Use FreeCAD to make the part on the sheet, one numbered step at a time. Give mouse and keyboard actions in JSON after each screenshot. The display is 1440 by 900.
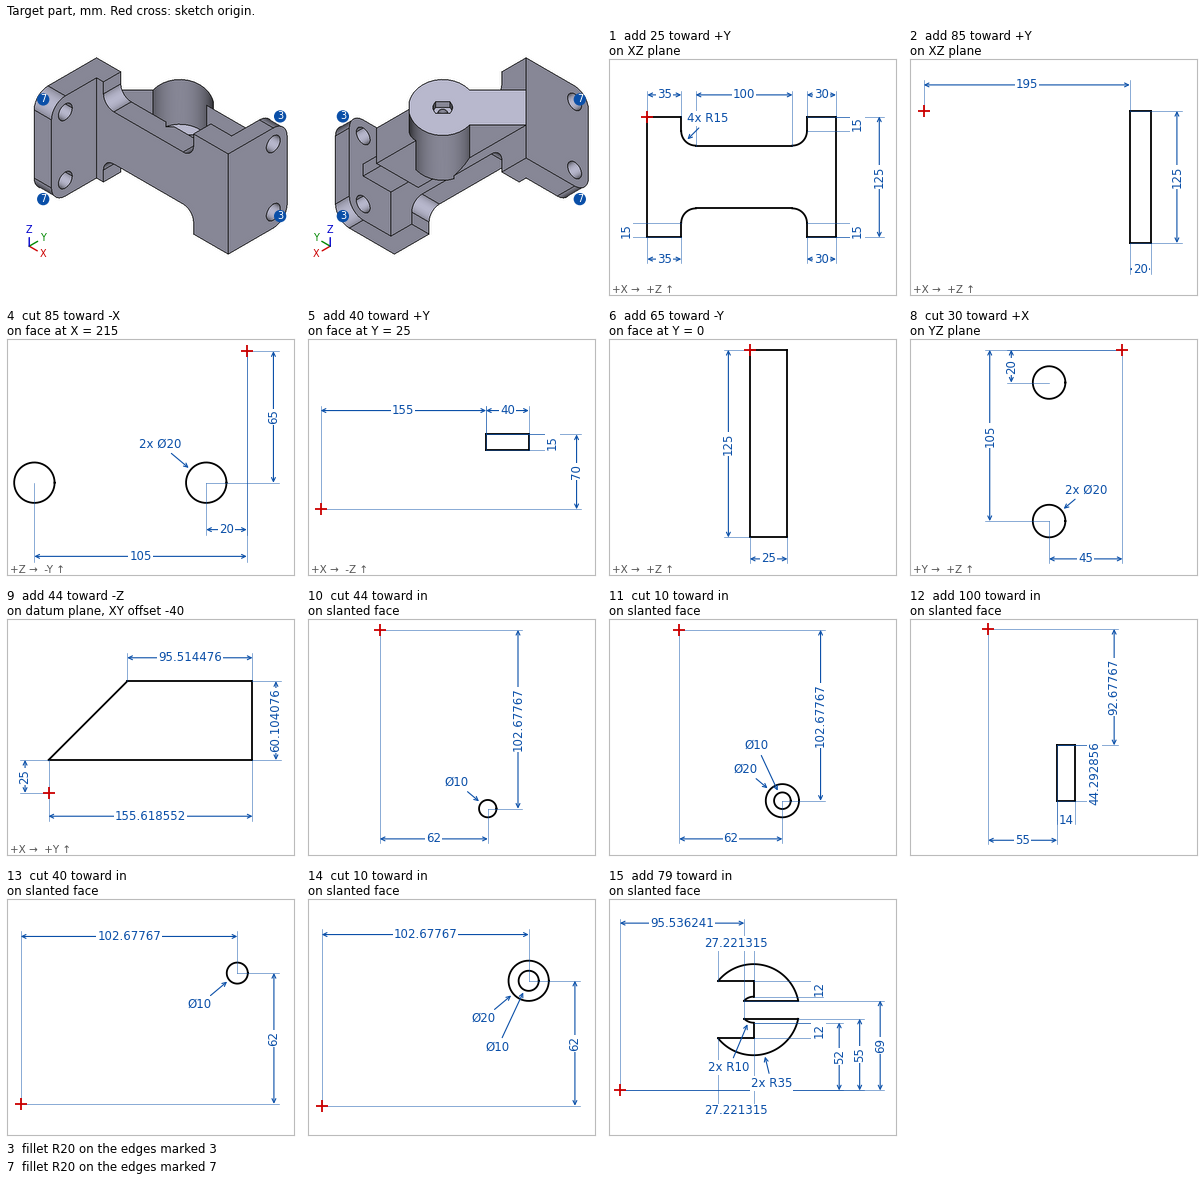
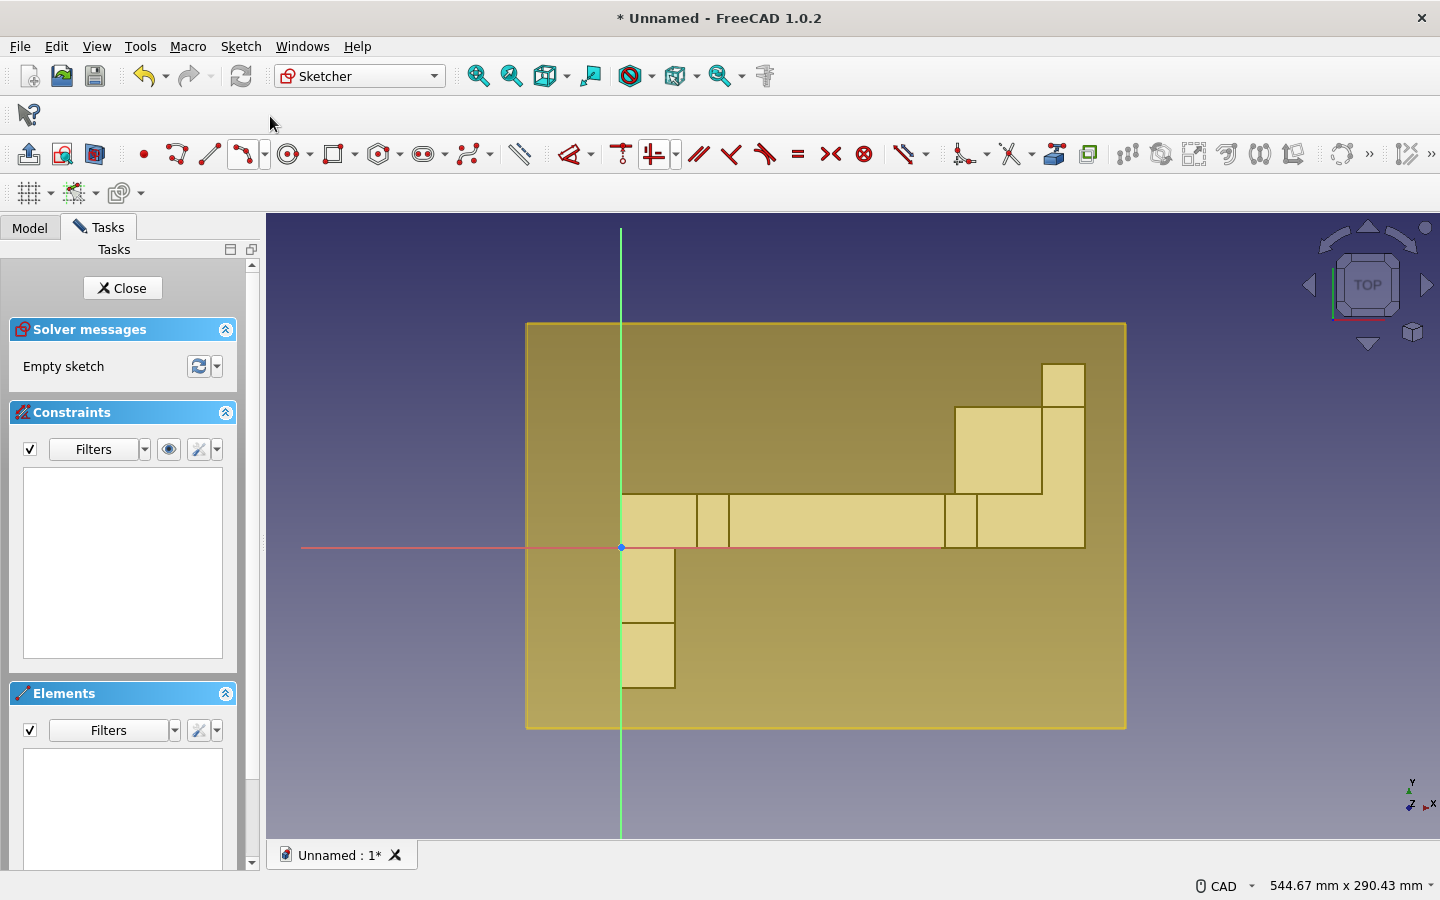
{"action": "scroll", "coordinate": [793, 399], "scroll_direction": "up", "scroll_amount": 4}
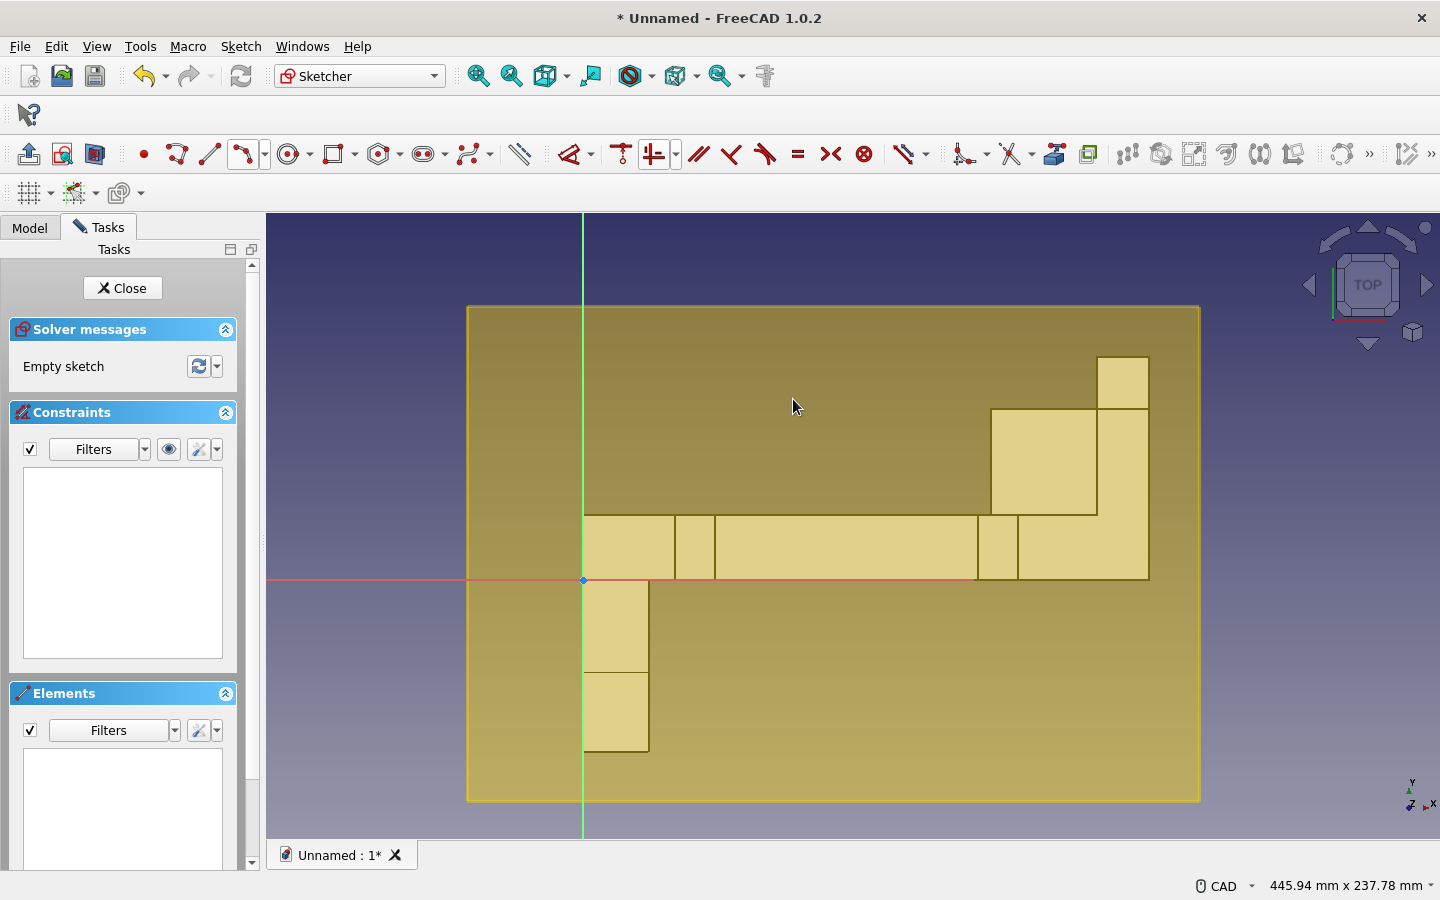
{"action": "left_click", "coordinate": [177, 154]}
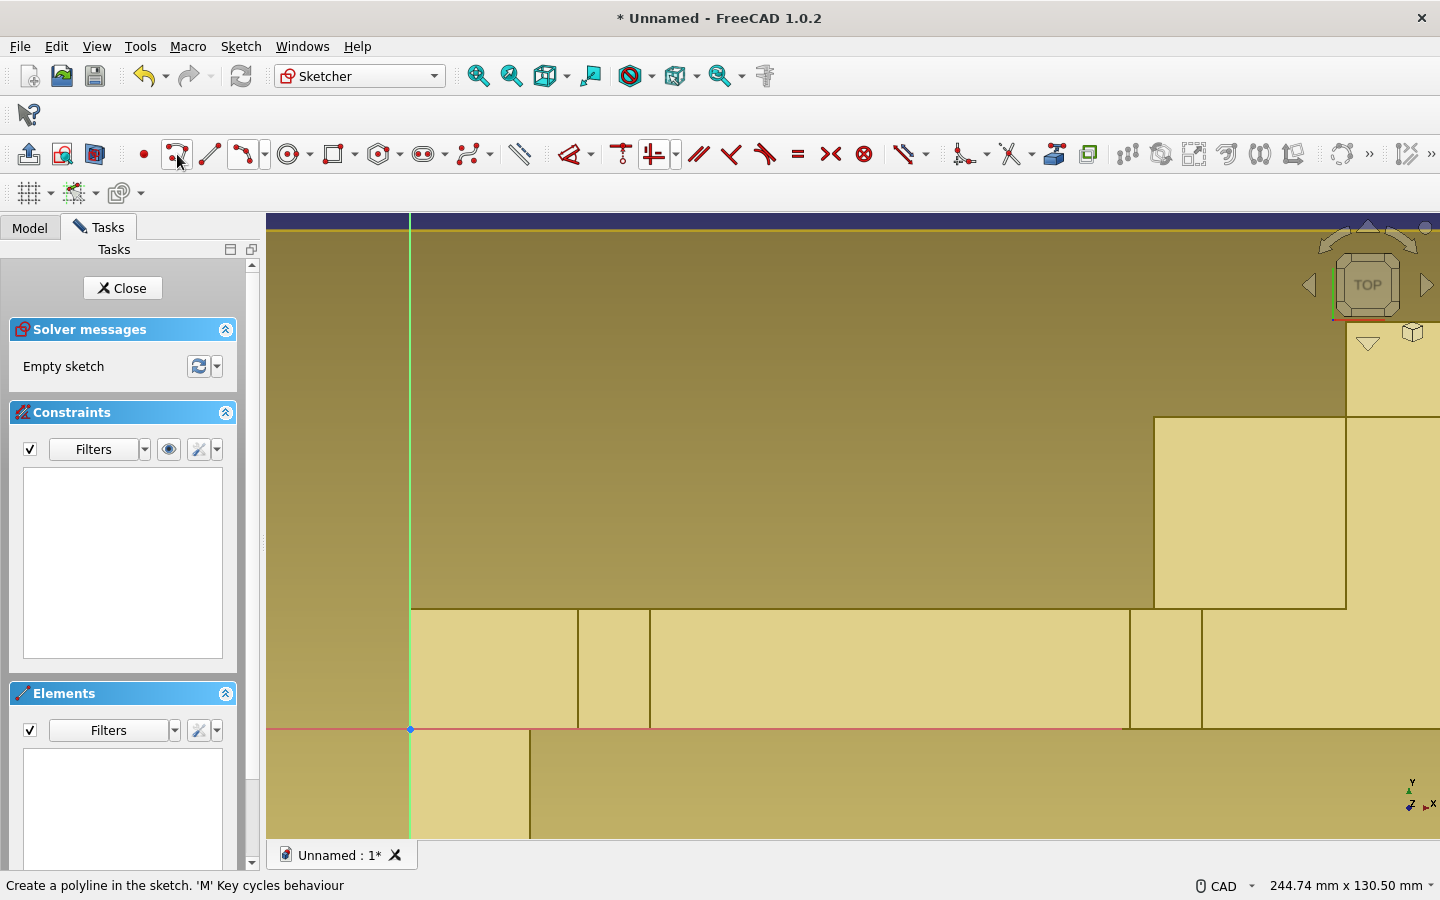
{"action": "left_click", "coordinate": [410, 609]}
{"action": "left_click", "coordinate": [1157, 609]}
{"action": "left_click", "coordinate": [1157, 321]}
{"action": "left_click", "coordinate": [699, 321]}
{"action": "left_click", "coordinate": [410, 610]}
{"action": "key", "text": "Escape"}
{"action": "key", "text": "Escape"}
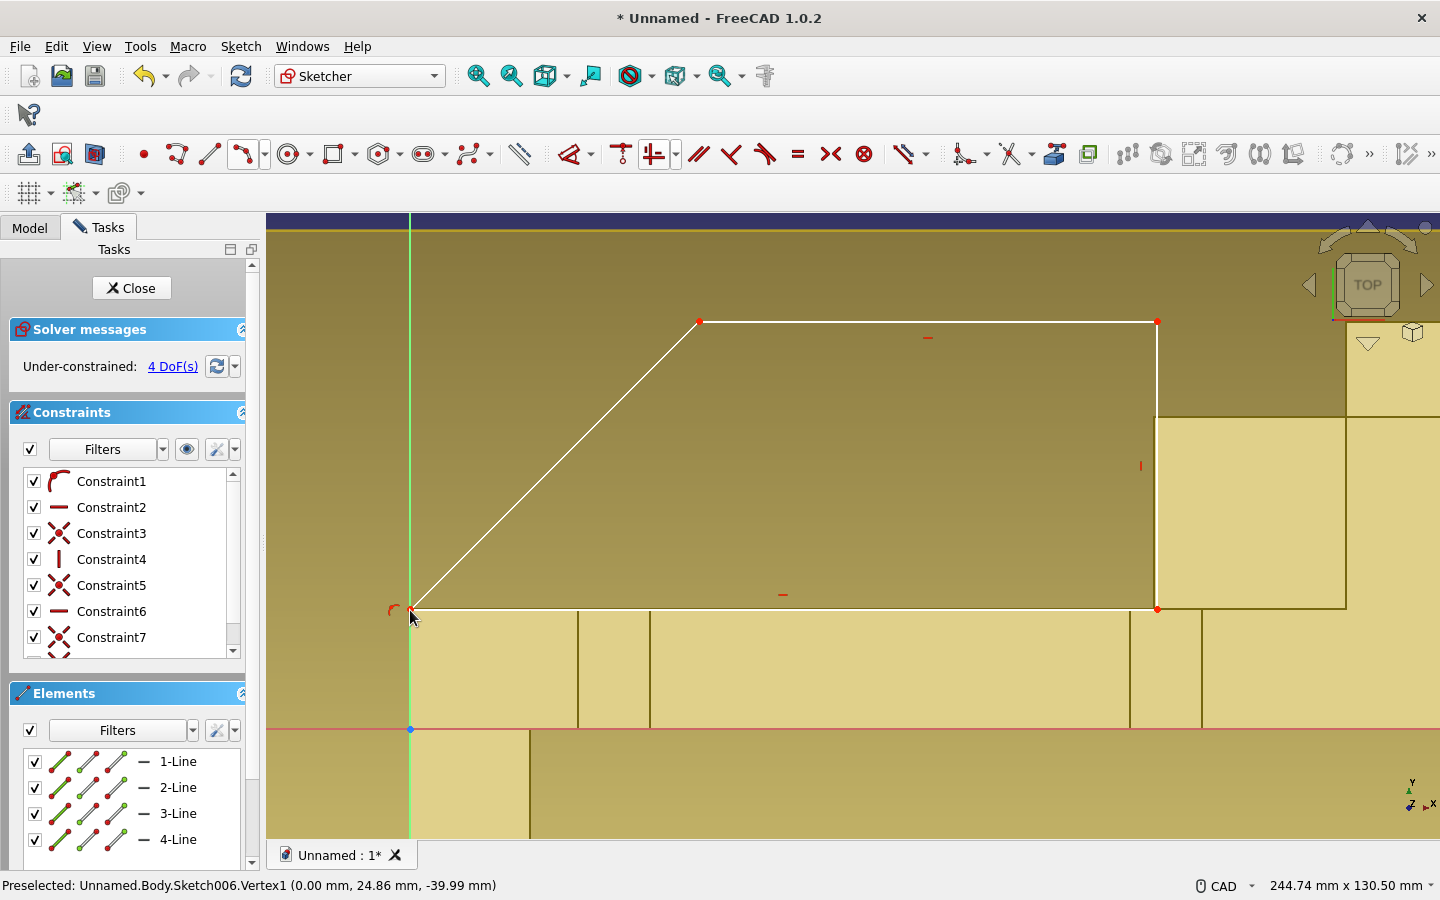
{"action": "left_click", "coordinate": [568, 154]}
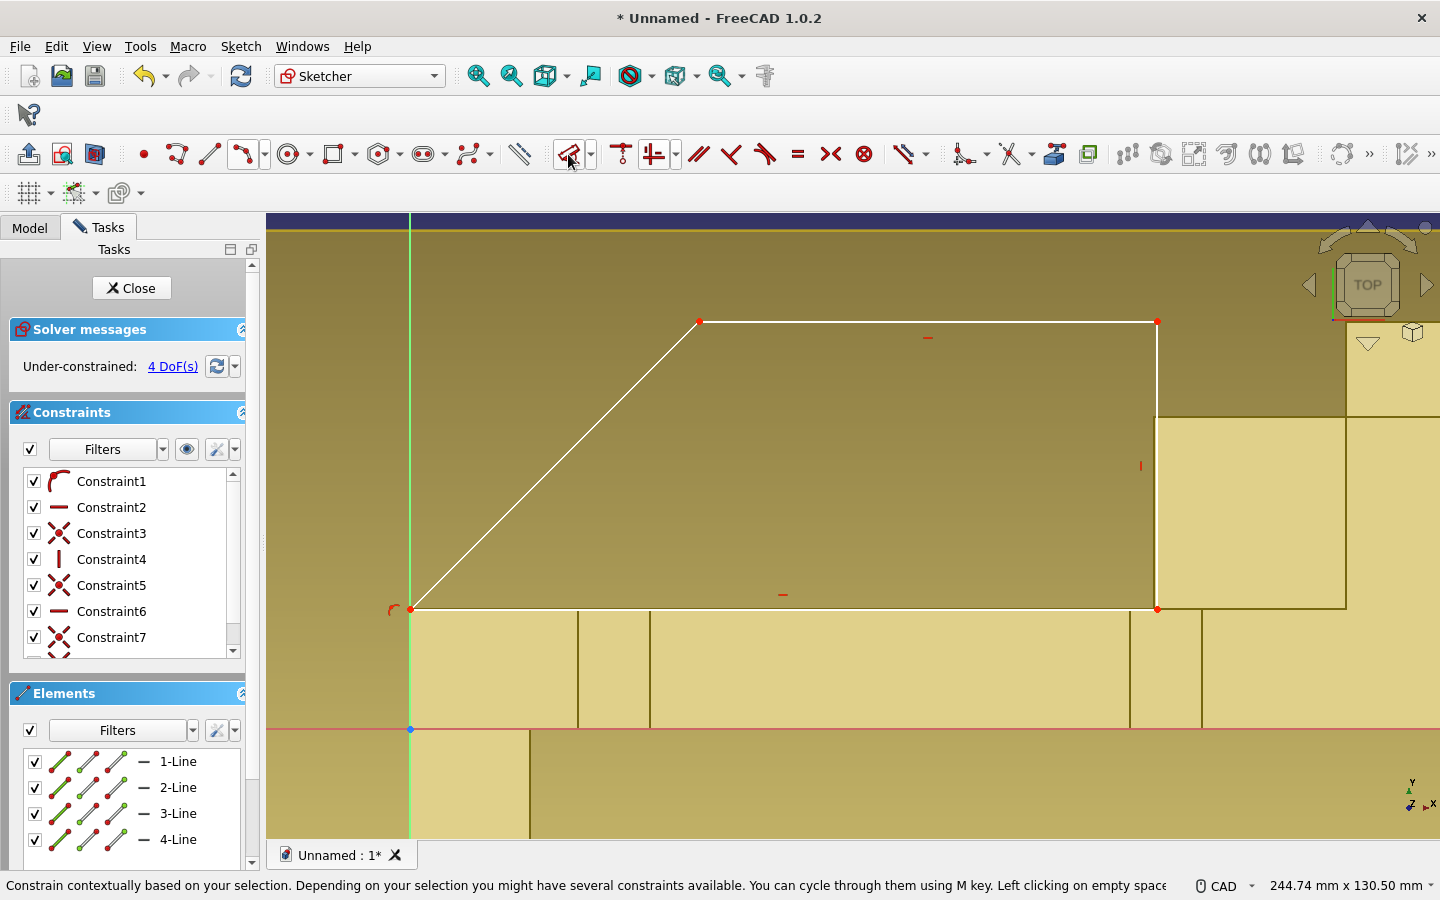
{"action": "left_click", "coordinate": [410, 610]}
{"action": "left_click", "coordinate": [376, 670]}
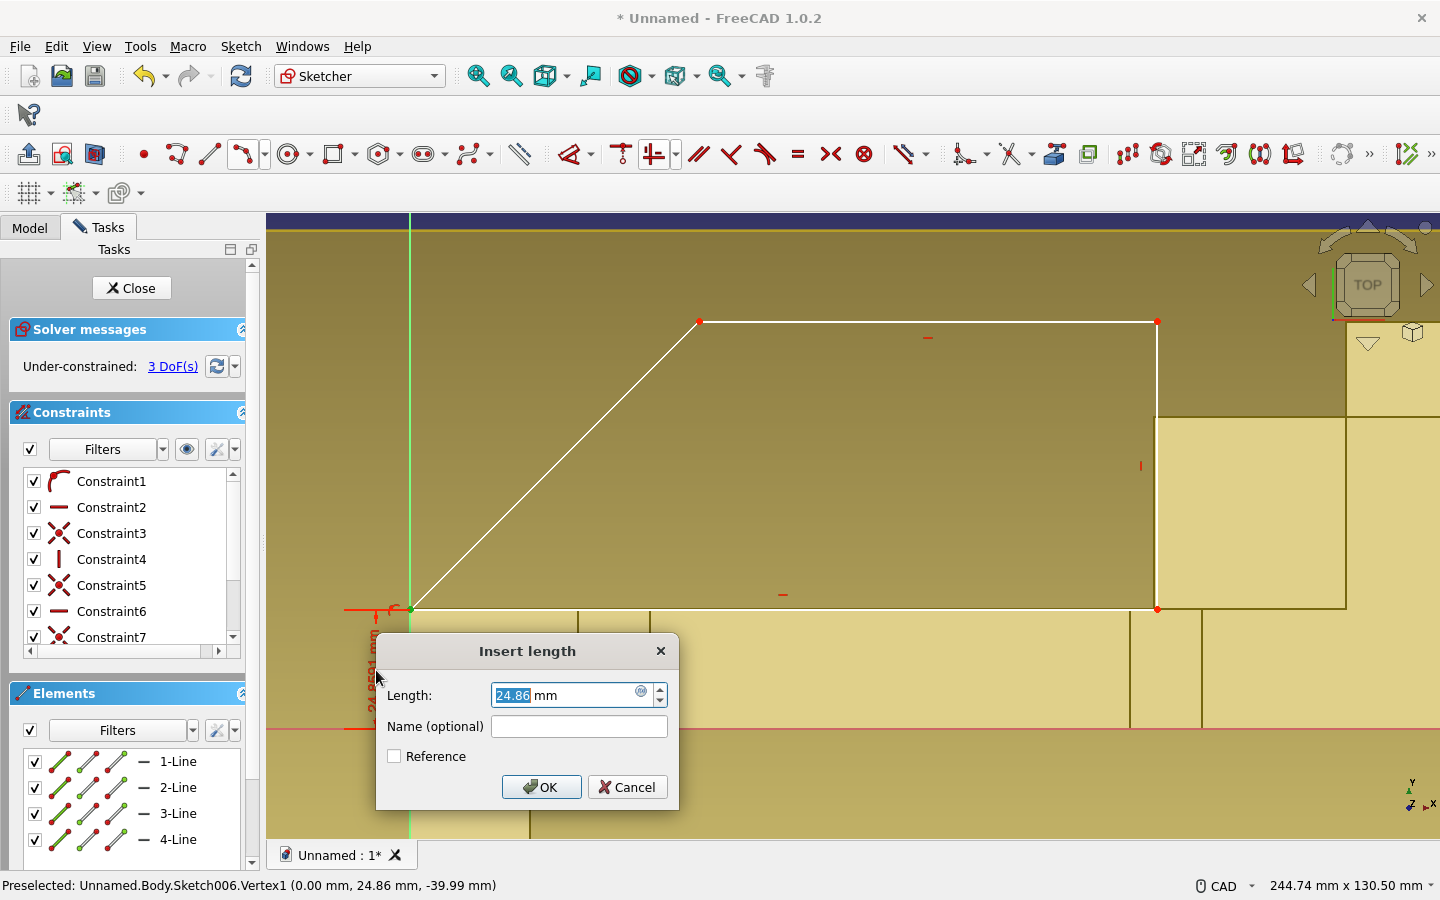
{"action": "type", "text": "25"}
{"action": "key", "text": "Return"}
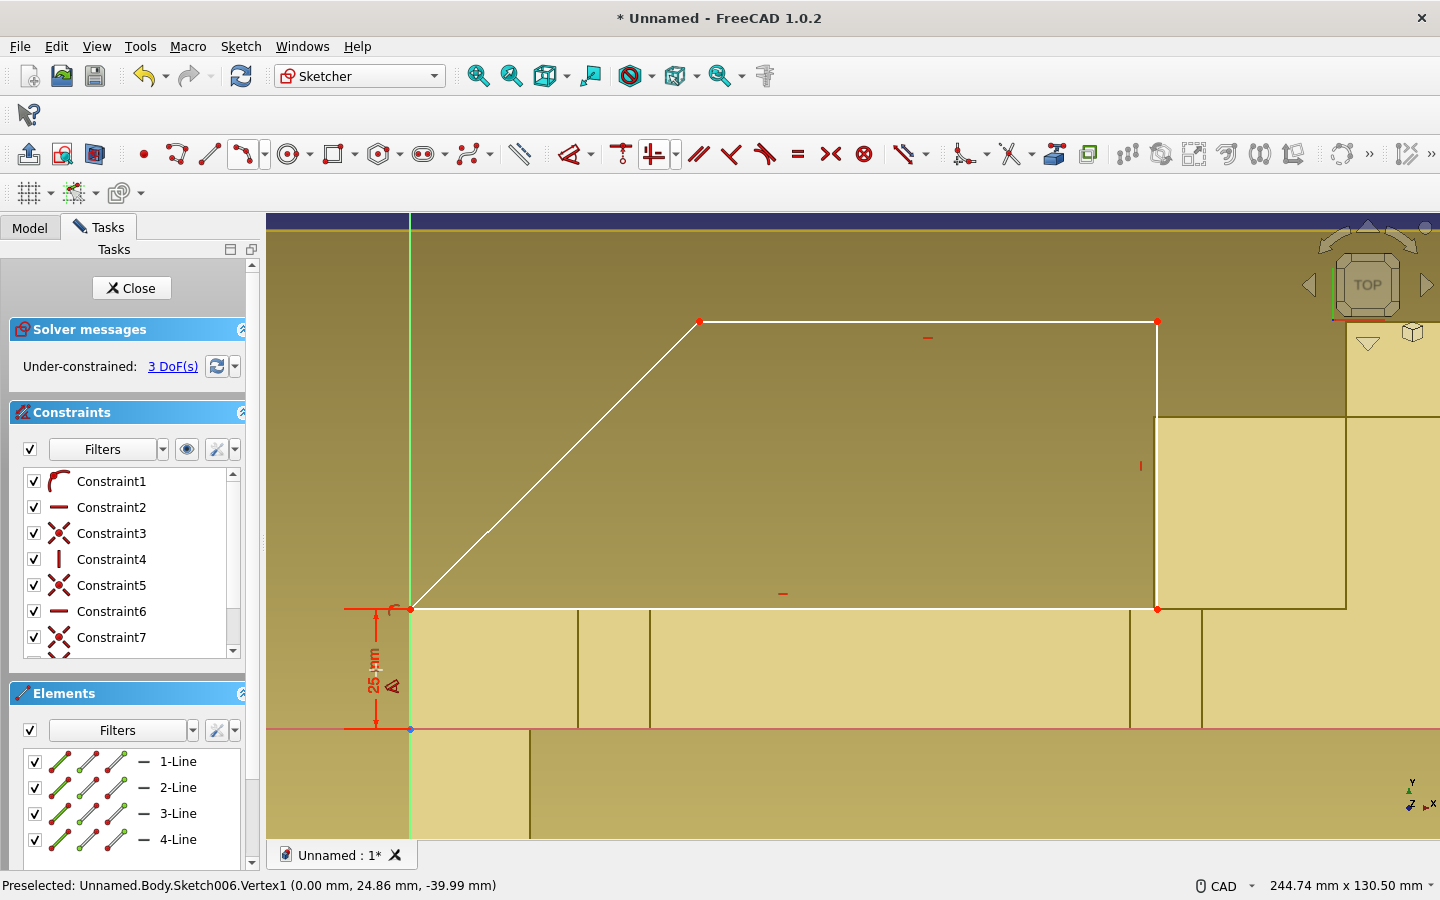
{"action": "left_click", "coordinate": [1157, 523]}
{"action": "left_click", "coordinate": [1191, 466]}